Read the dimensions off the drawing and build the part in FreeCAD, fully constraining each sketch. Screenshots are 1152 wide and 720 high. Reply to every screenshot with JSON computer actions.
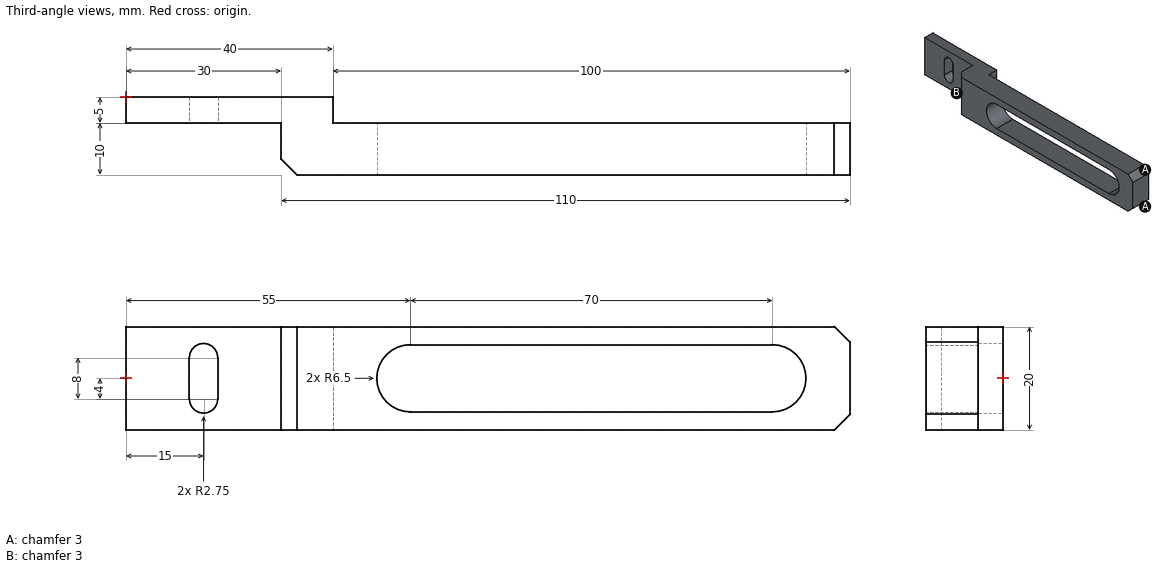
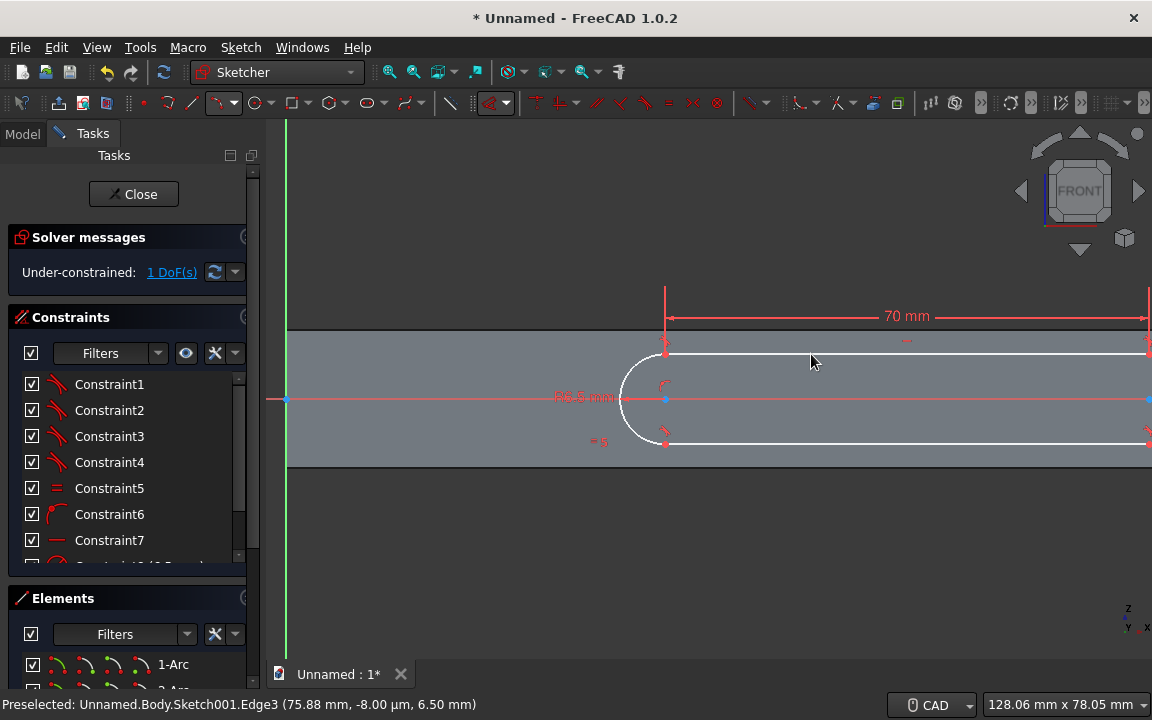
{"action": "left_click", "coordinate": [665, 354]}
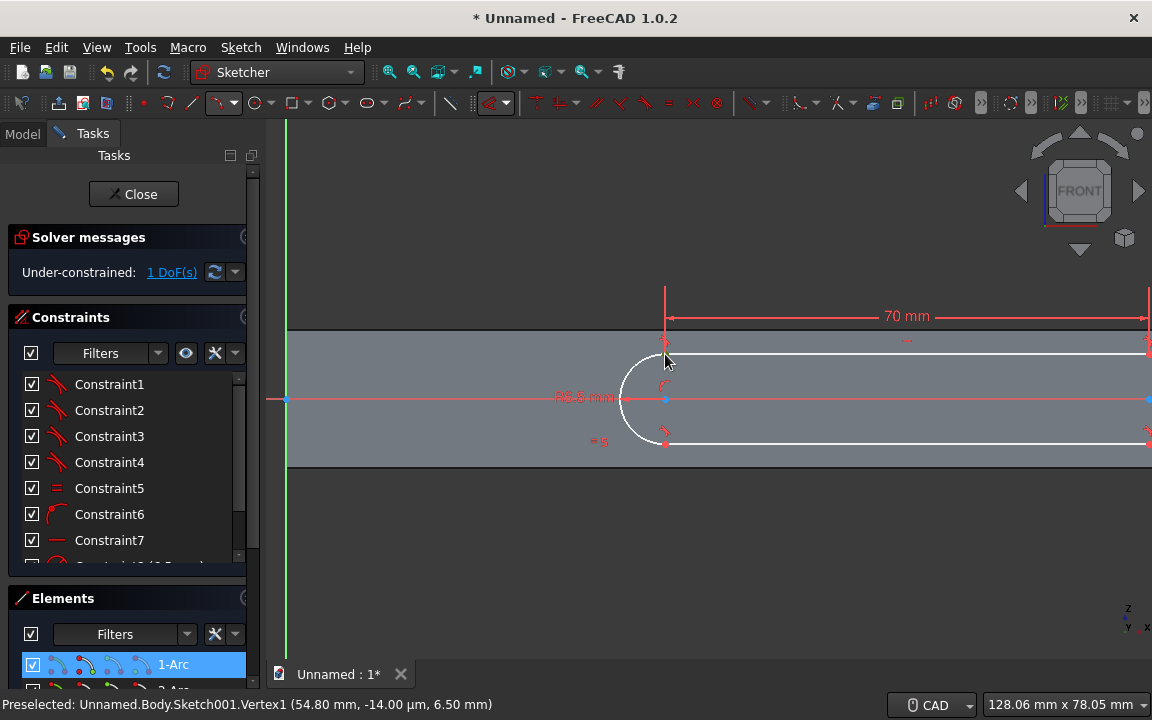
{"action": "key", "text": "l"}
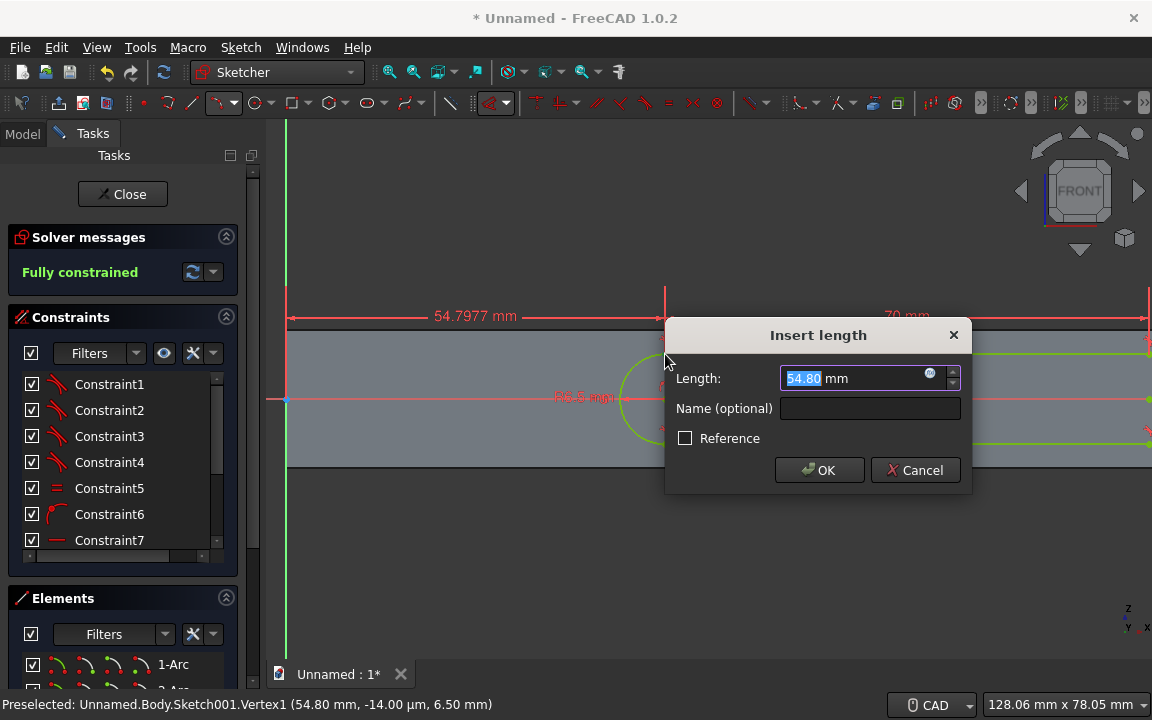
{"action": "type", "text": "55"}
{"action": "key", "text": "Return"}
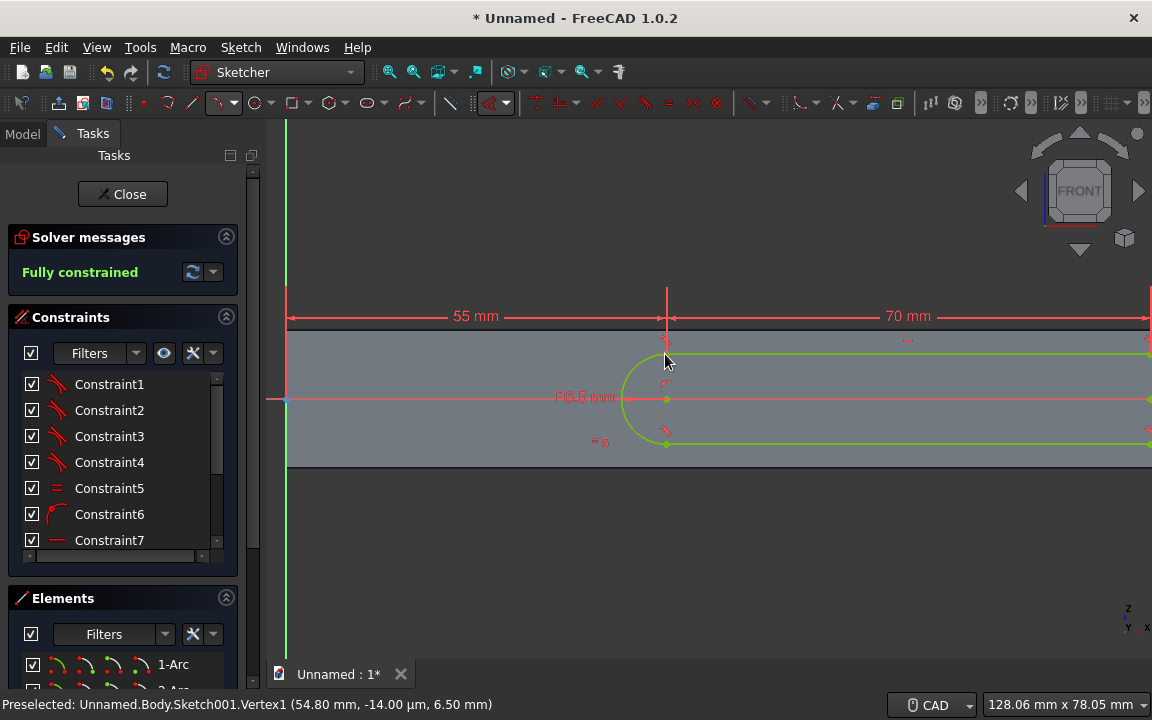
{"action": "left_click", "coordinate": [123, 194]}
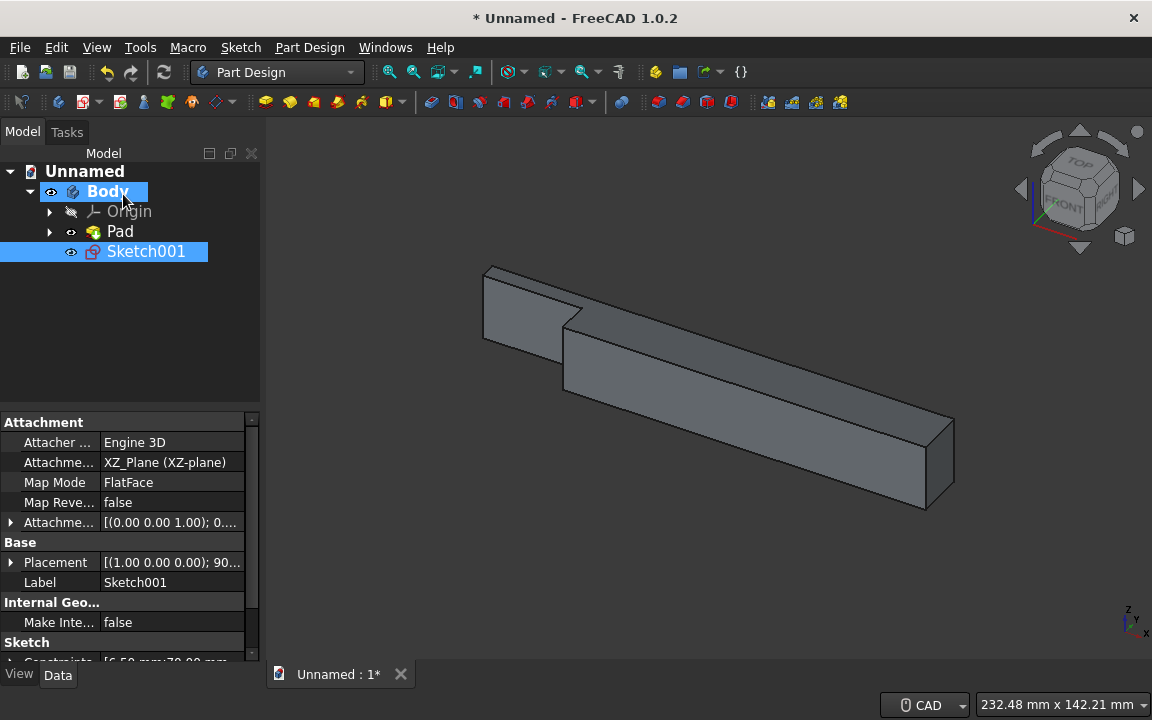
{"action": "left_click", "coordinate": [432, 102]}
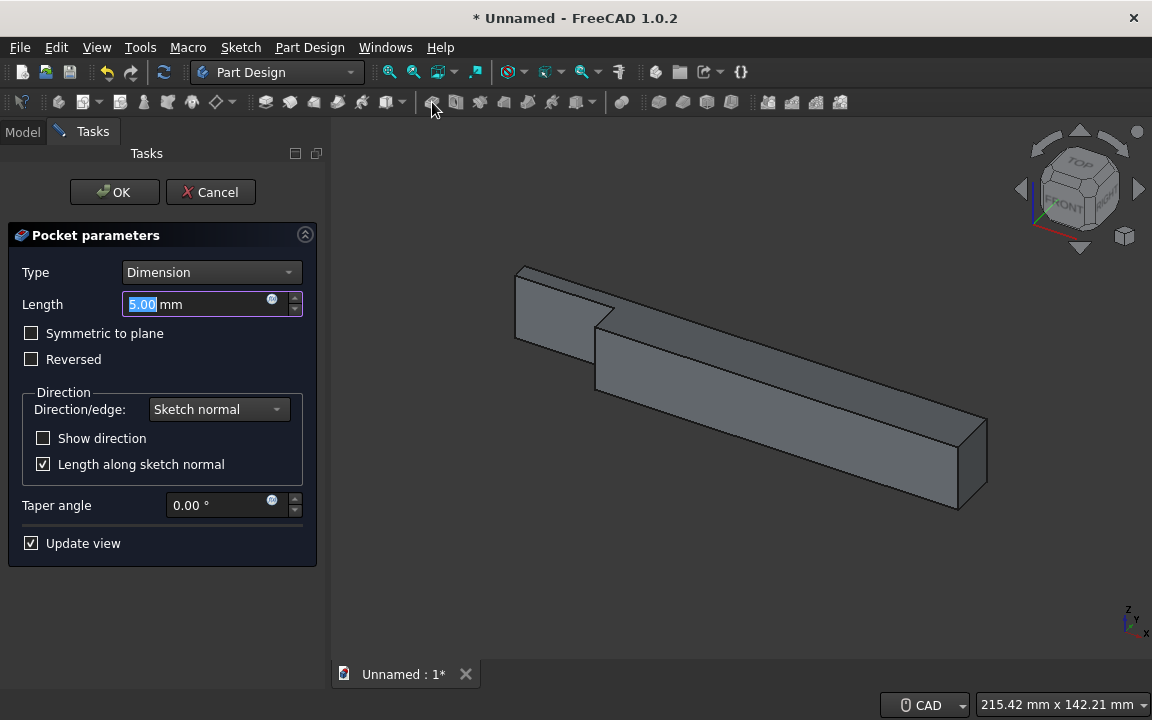
{"action": "left_click", "coordinate": [212, 272]}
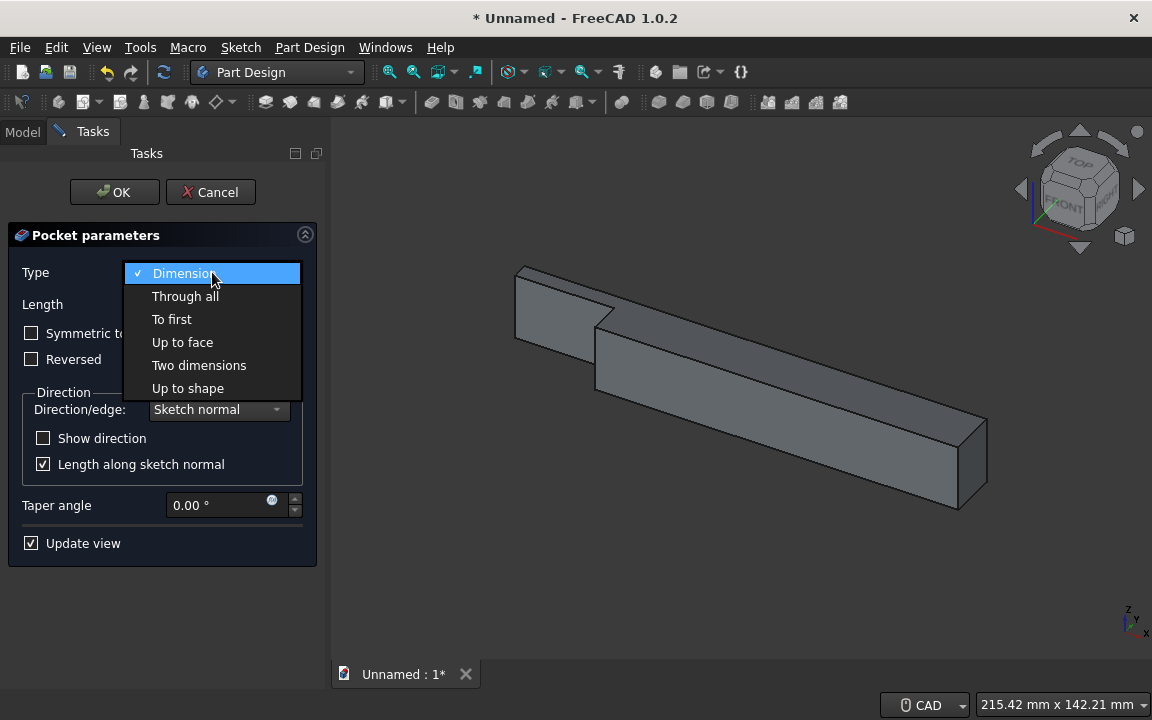
{"action": "left_click", "coordinate": [212, 296]}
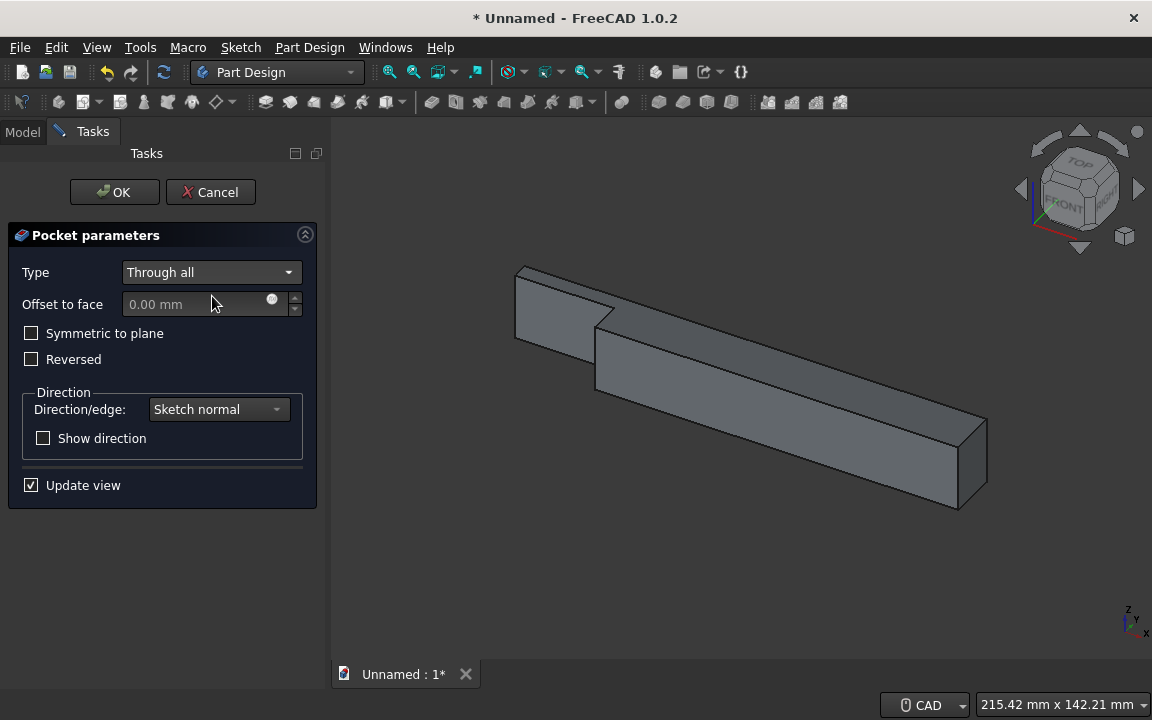
{"action": "left_click", "coordinate": [30, 359]}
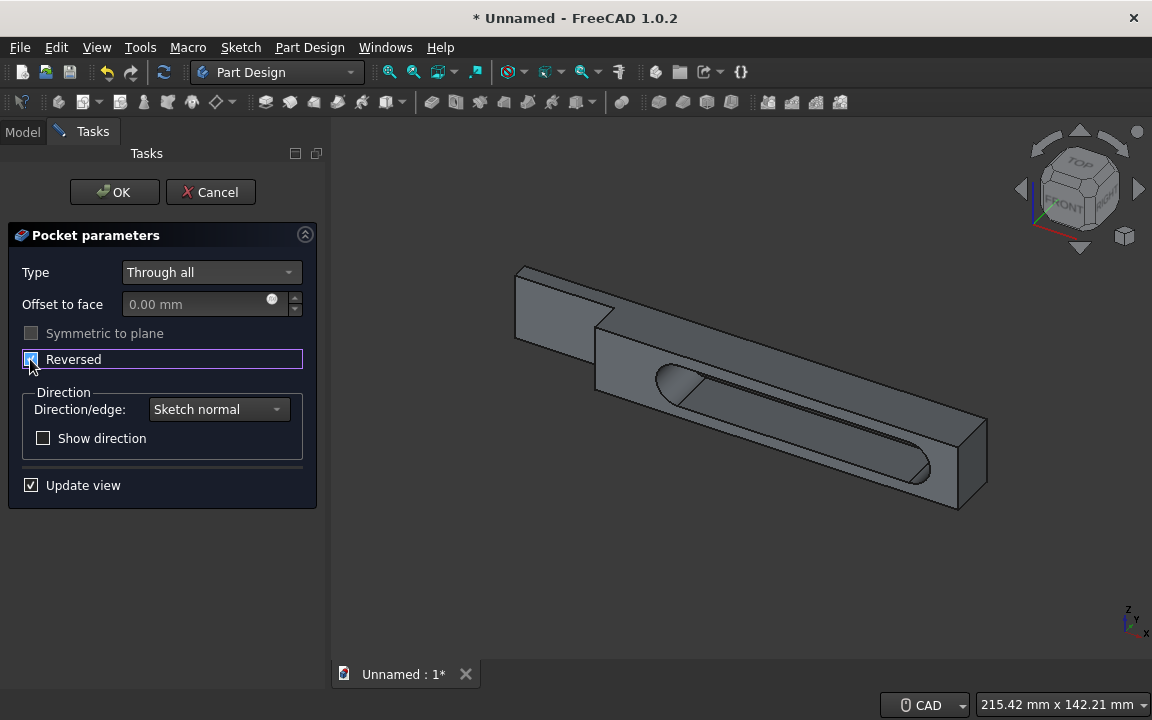
{"action": "left_click", "coordinate": [115, 192]}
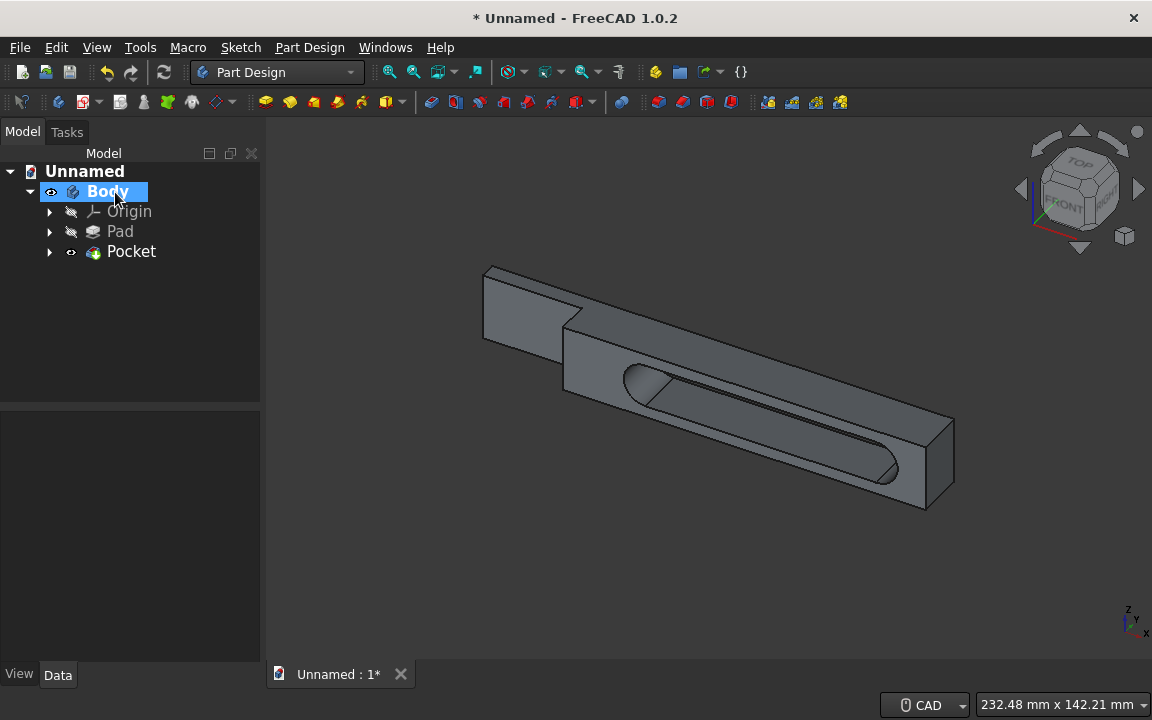
{"action": "key", "text": "4"}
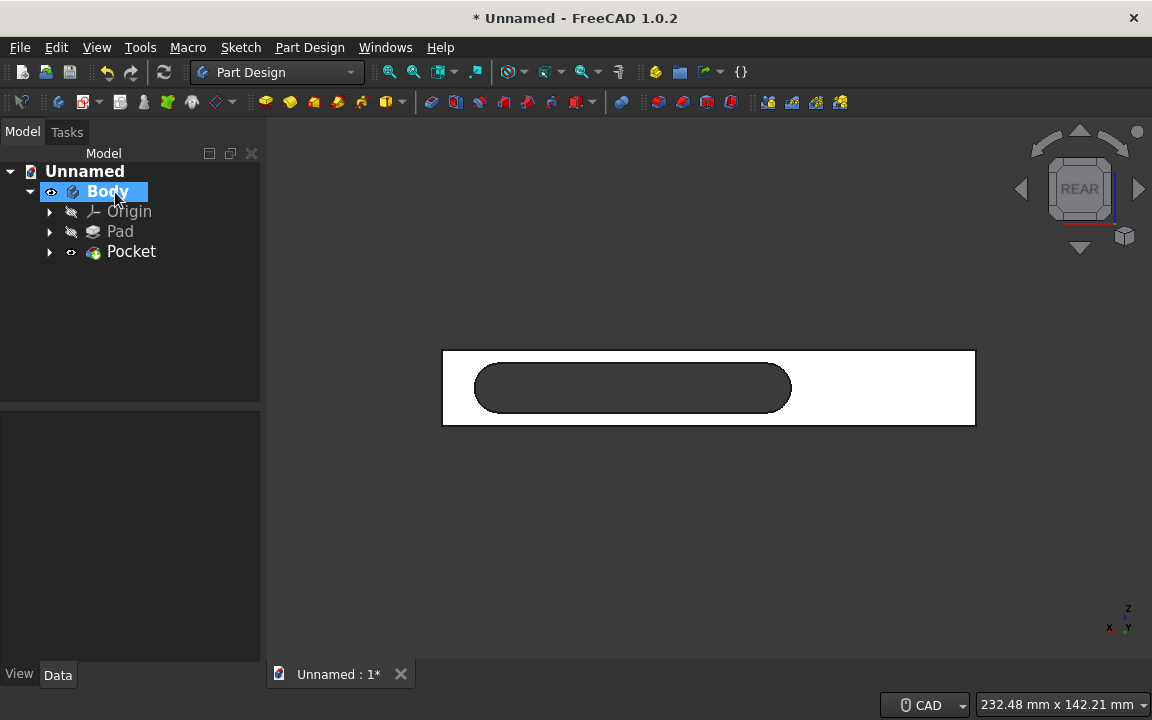
{"action": "left_click", "coordinate": [861, 387]}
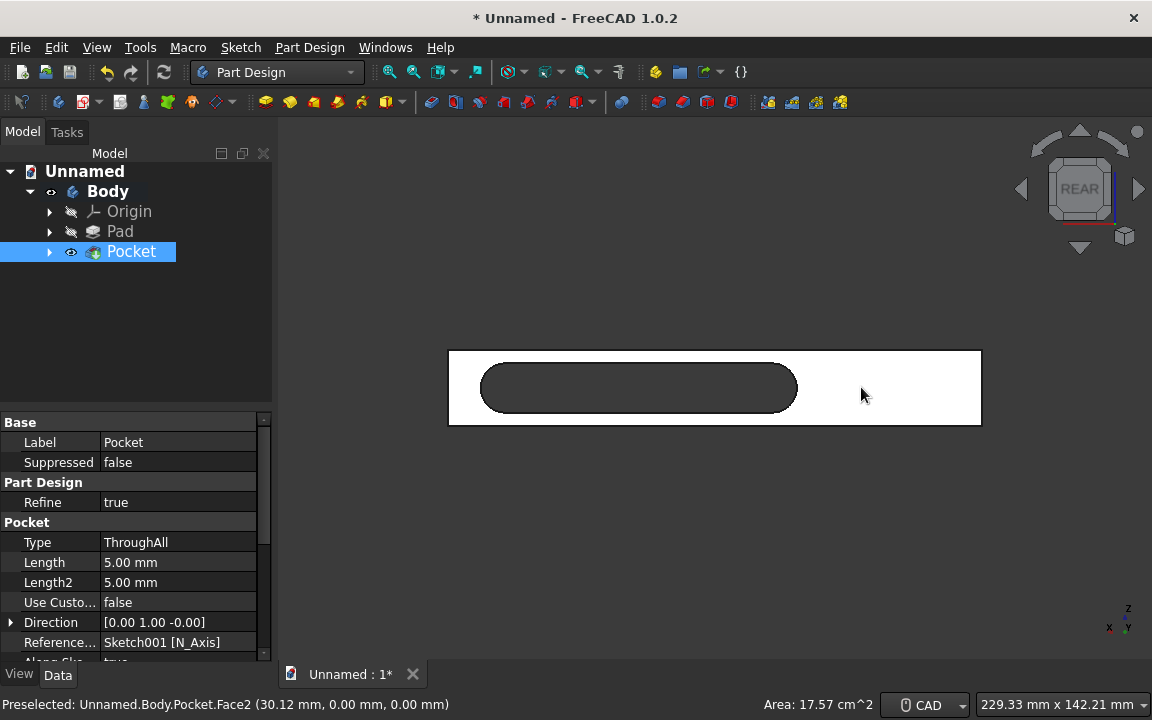
{"action": "left_click", "coordinate": [84, 102]}